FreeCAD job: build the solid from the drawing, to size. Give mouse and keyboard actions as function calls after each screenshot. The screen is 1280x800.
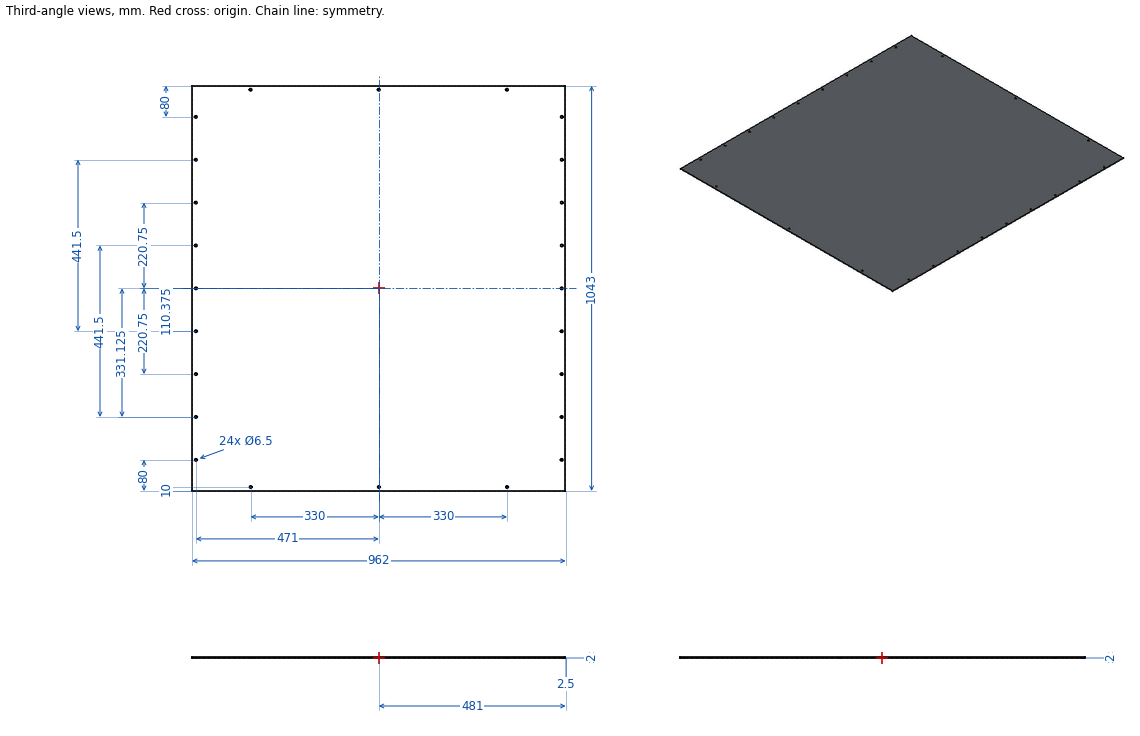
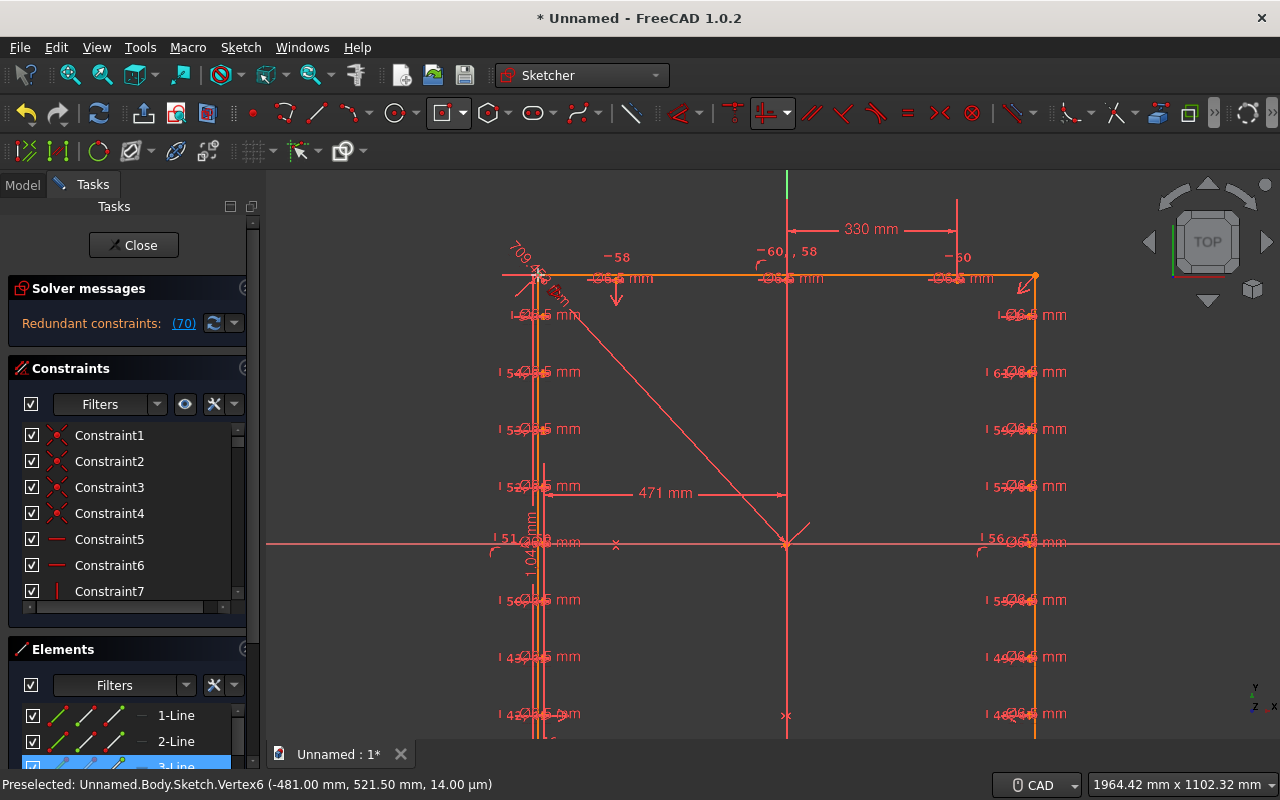
click(544, 317)
click(504, 296)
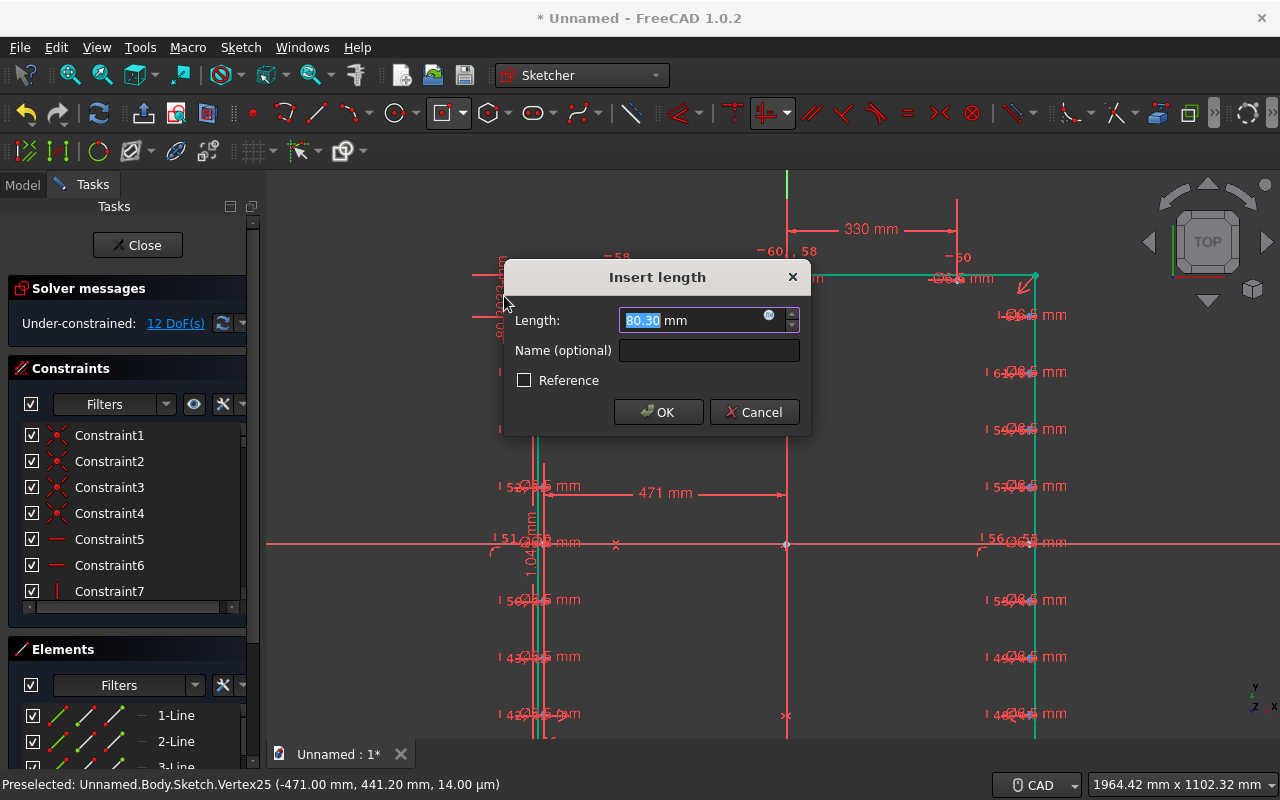
text(80)
key(Return)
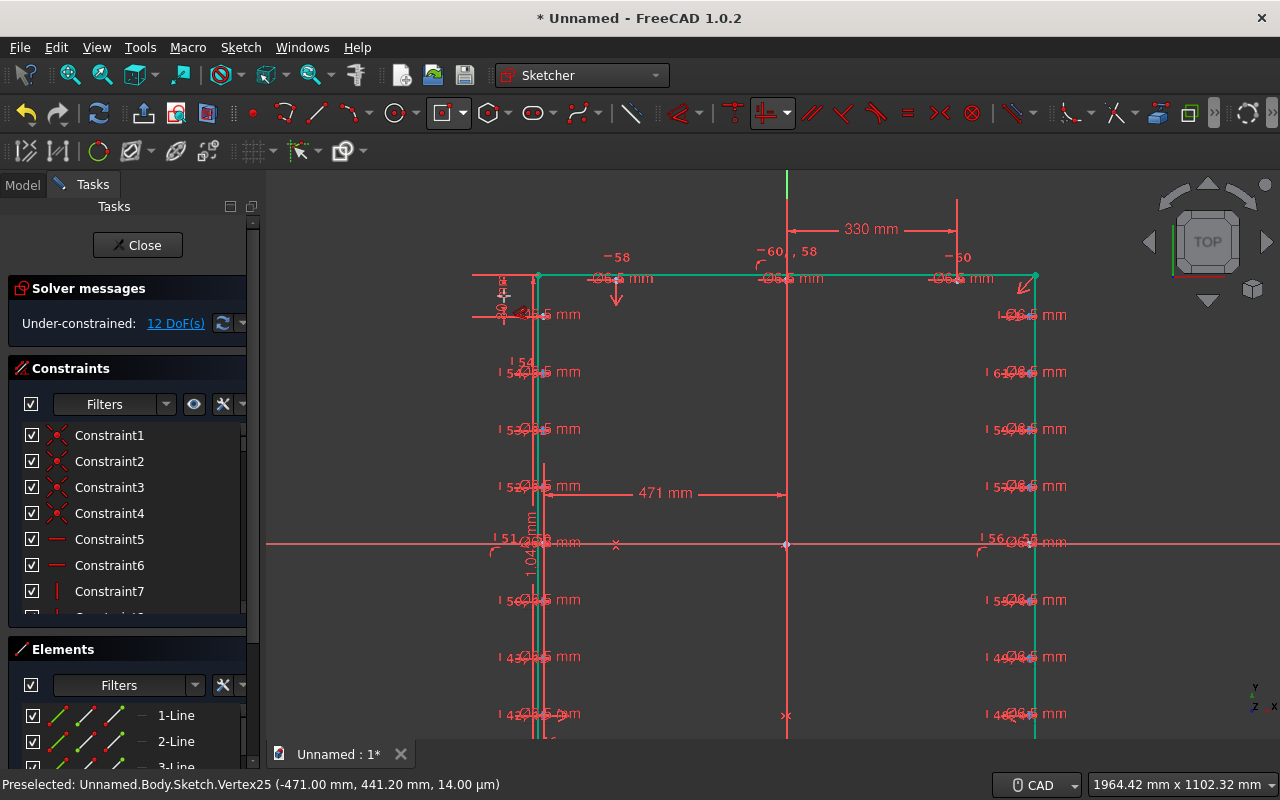
click(1035, 275)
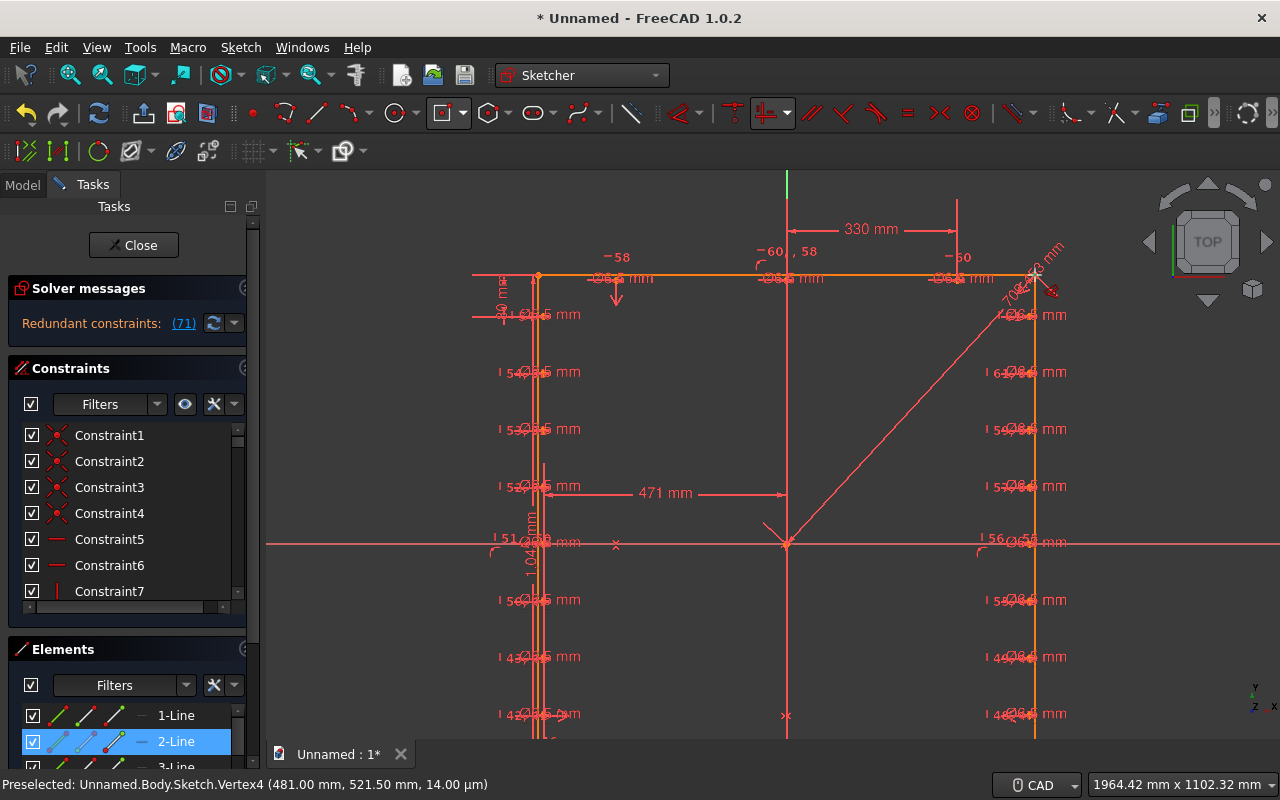
click(1030, 317)
click(1069, 296)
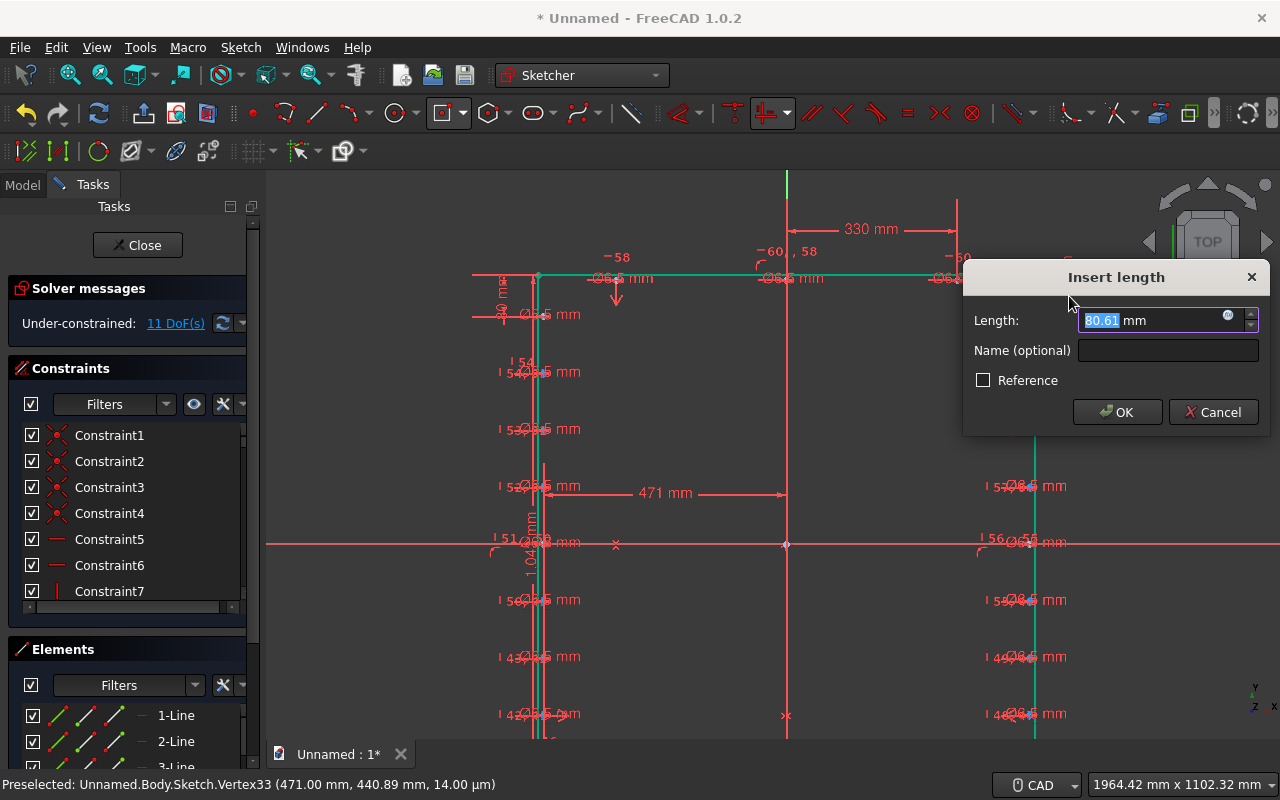
text(80)
key(Return)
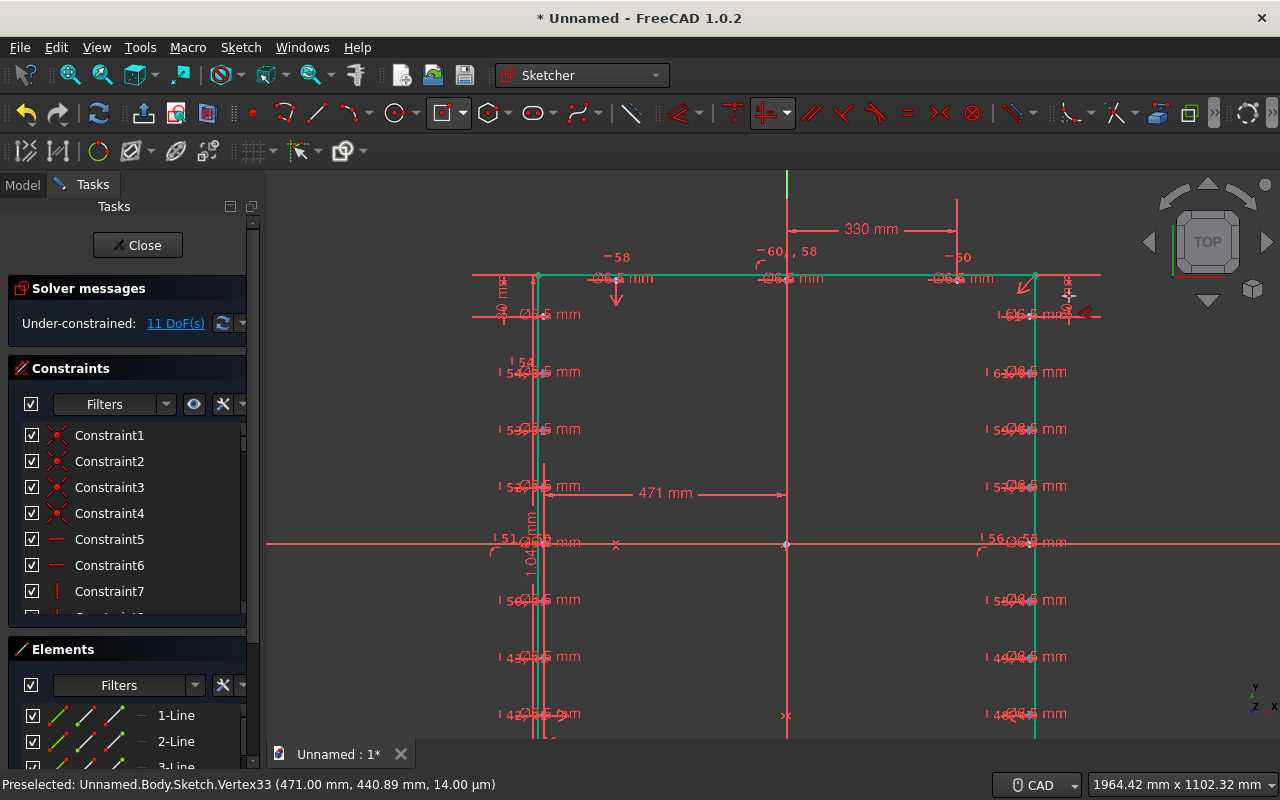
click(544, 659)
click(510, 601)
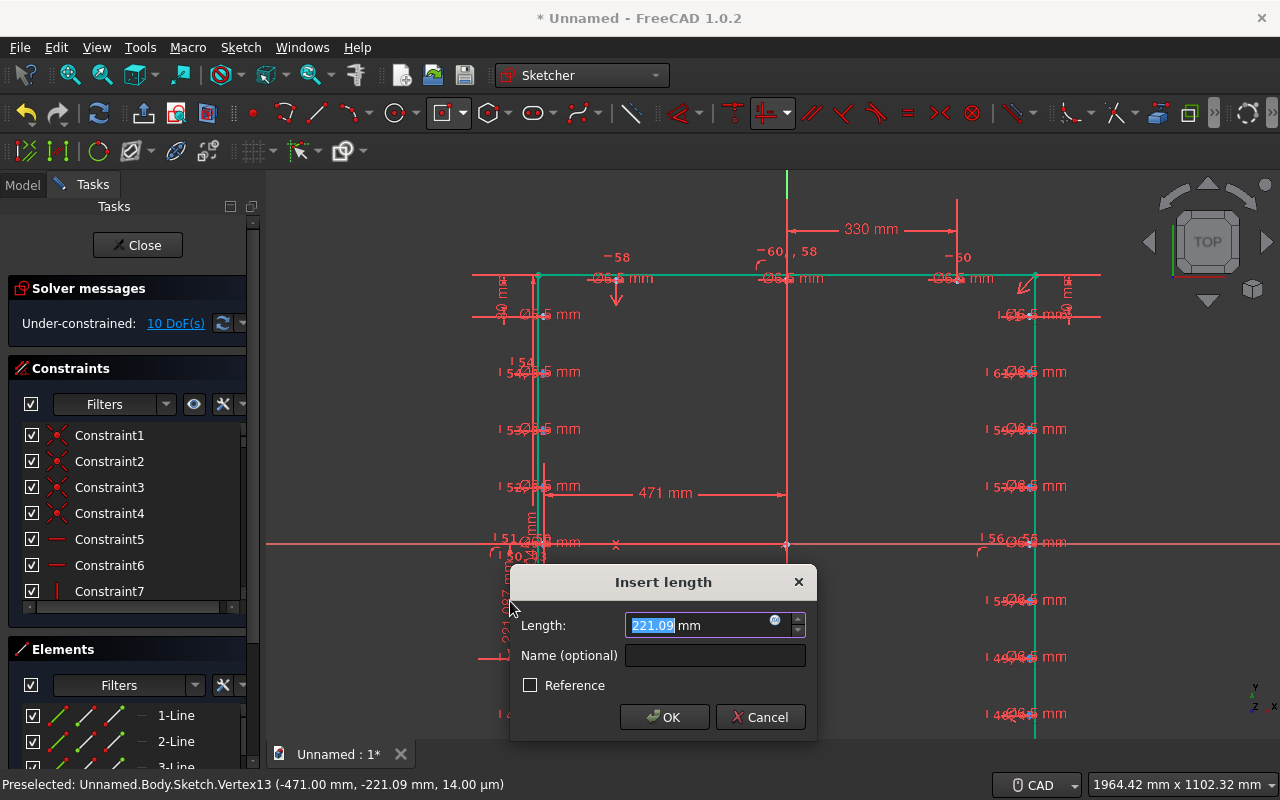
text(220.75)
key(Return)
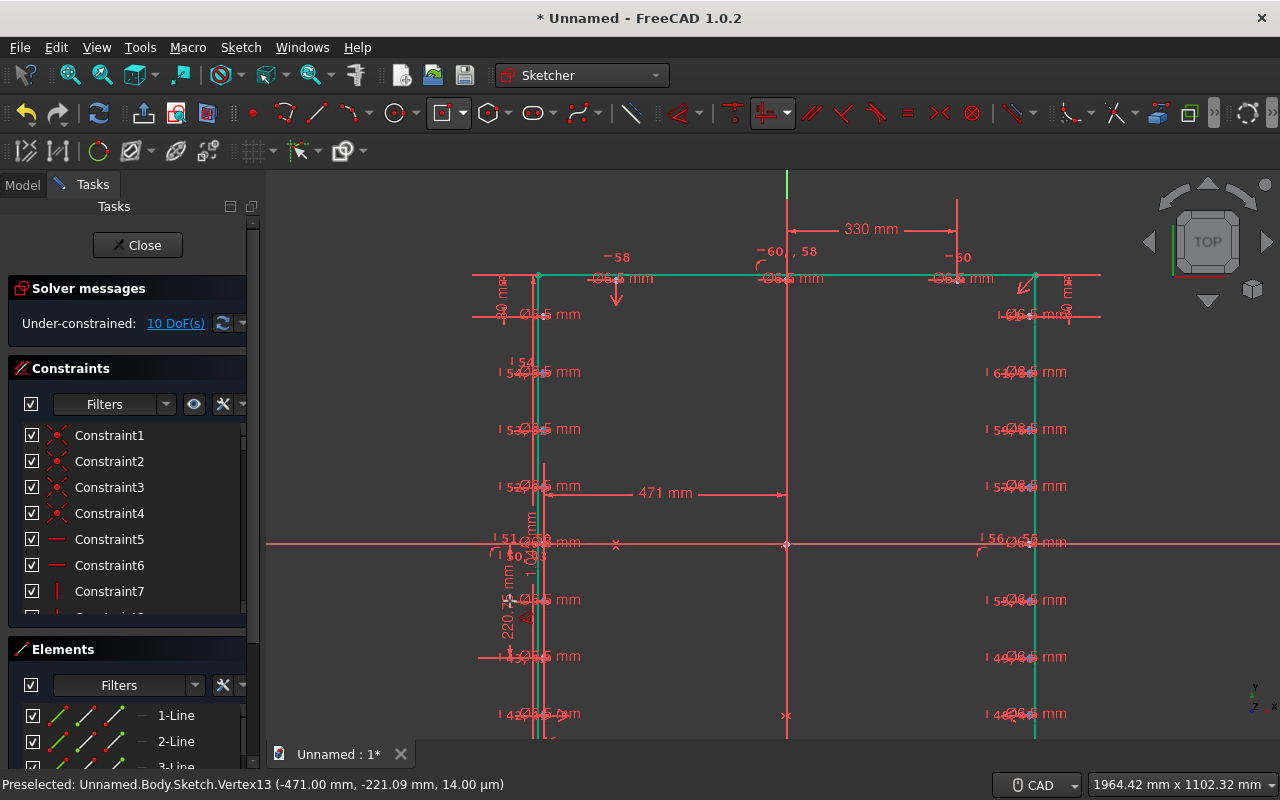
click(1030, 659)
click(1064, 602)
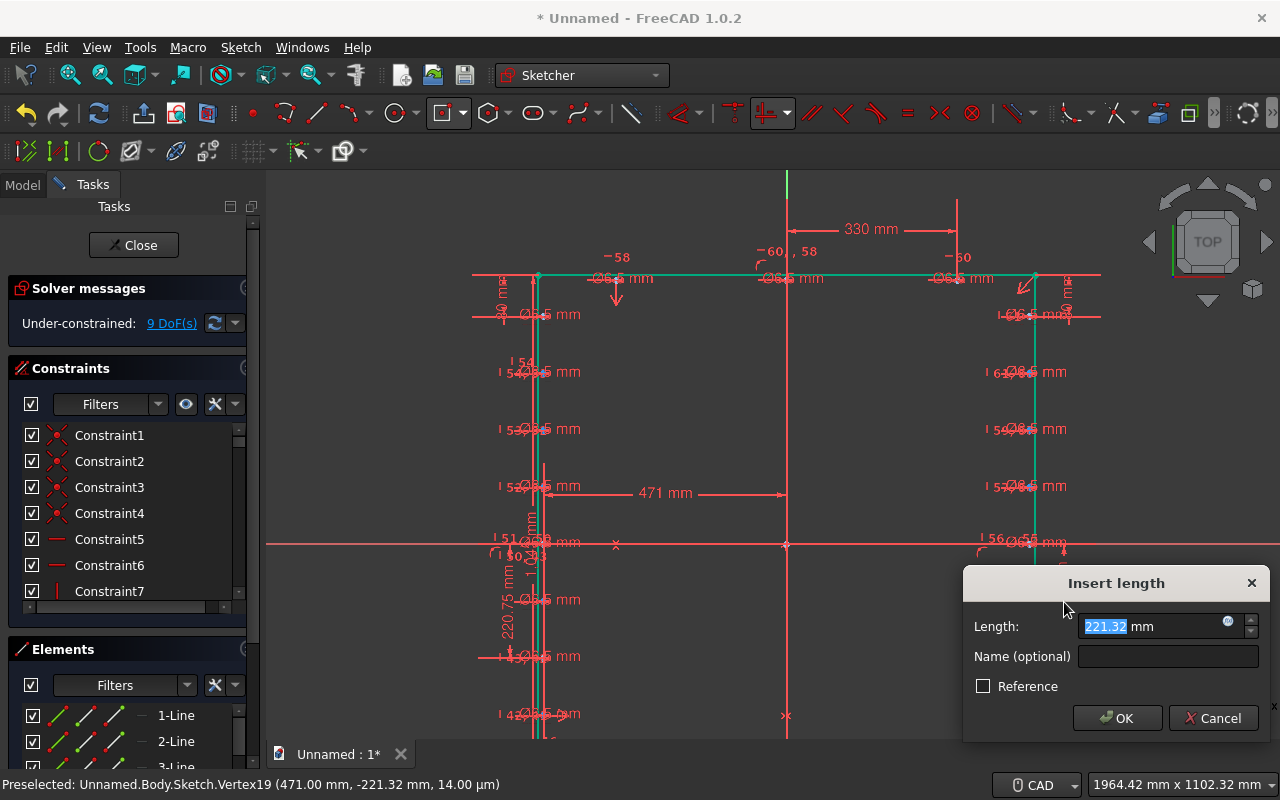
text(220.75)
key(Return)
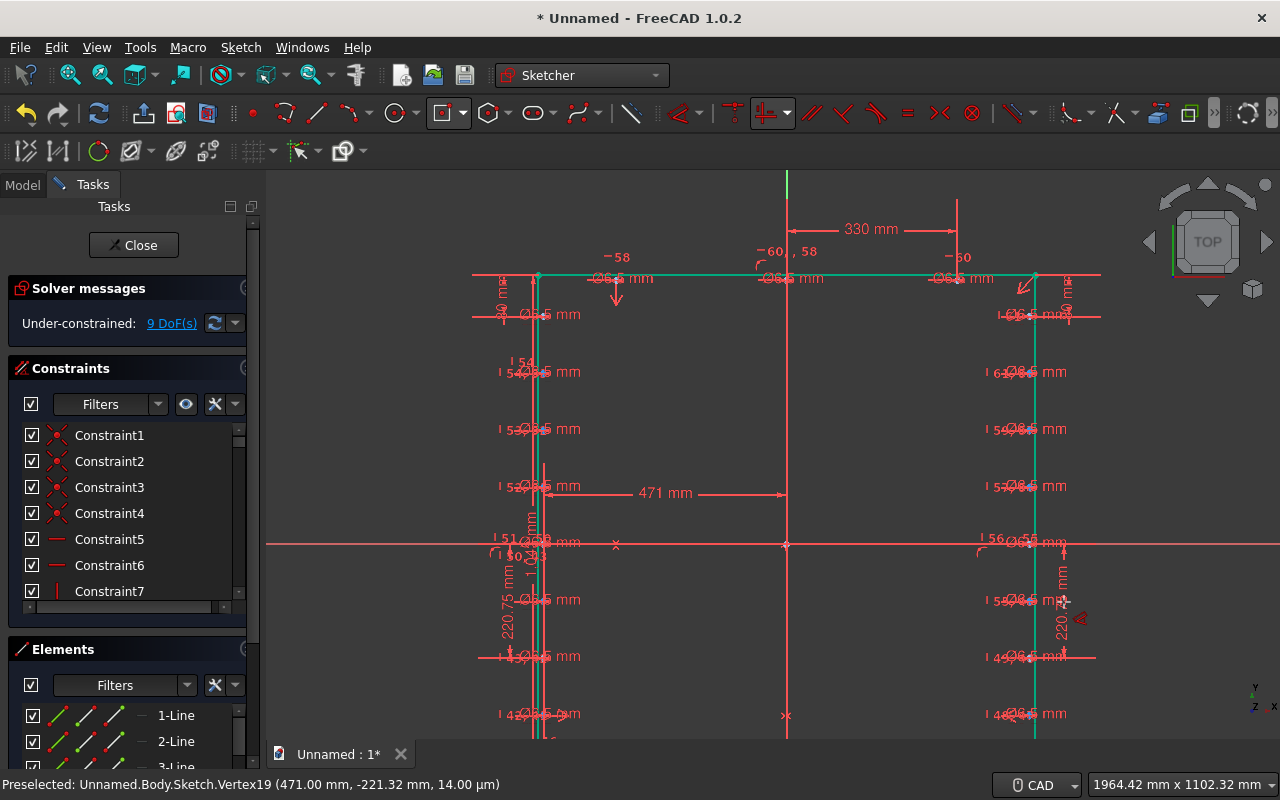
click(544, 431)
click(510, 488)